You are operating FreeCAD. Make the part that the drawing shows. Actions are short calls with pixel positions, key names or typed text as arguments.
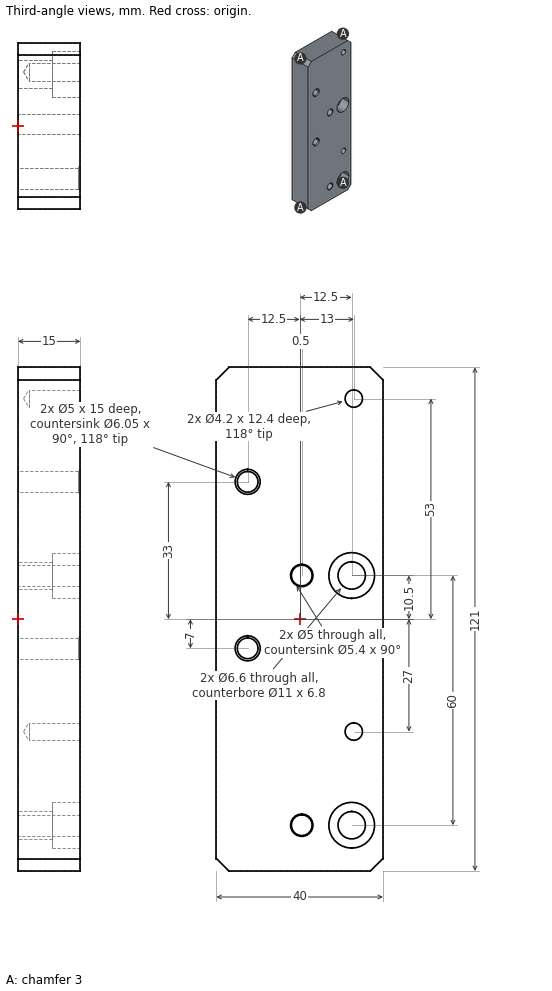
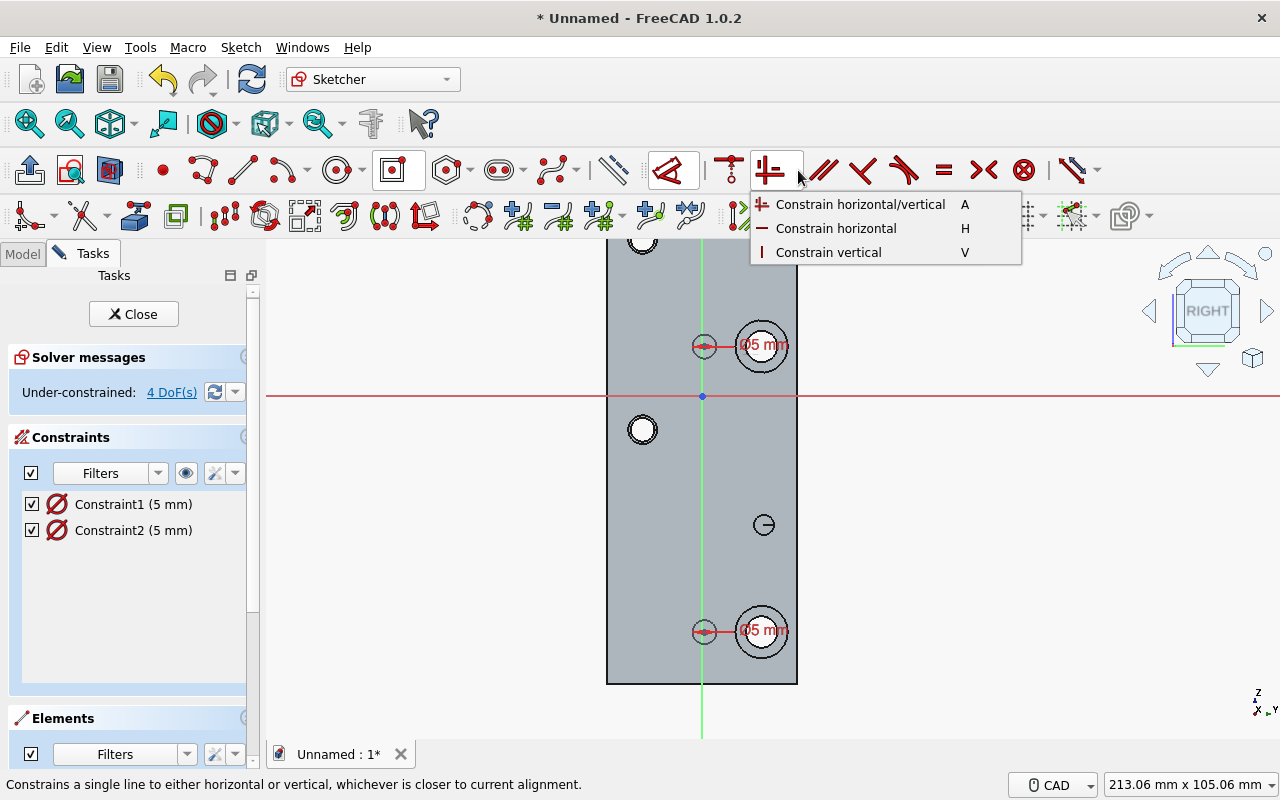
click(886, 252)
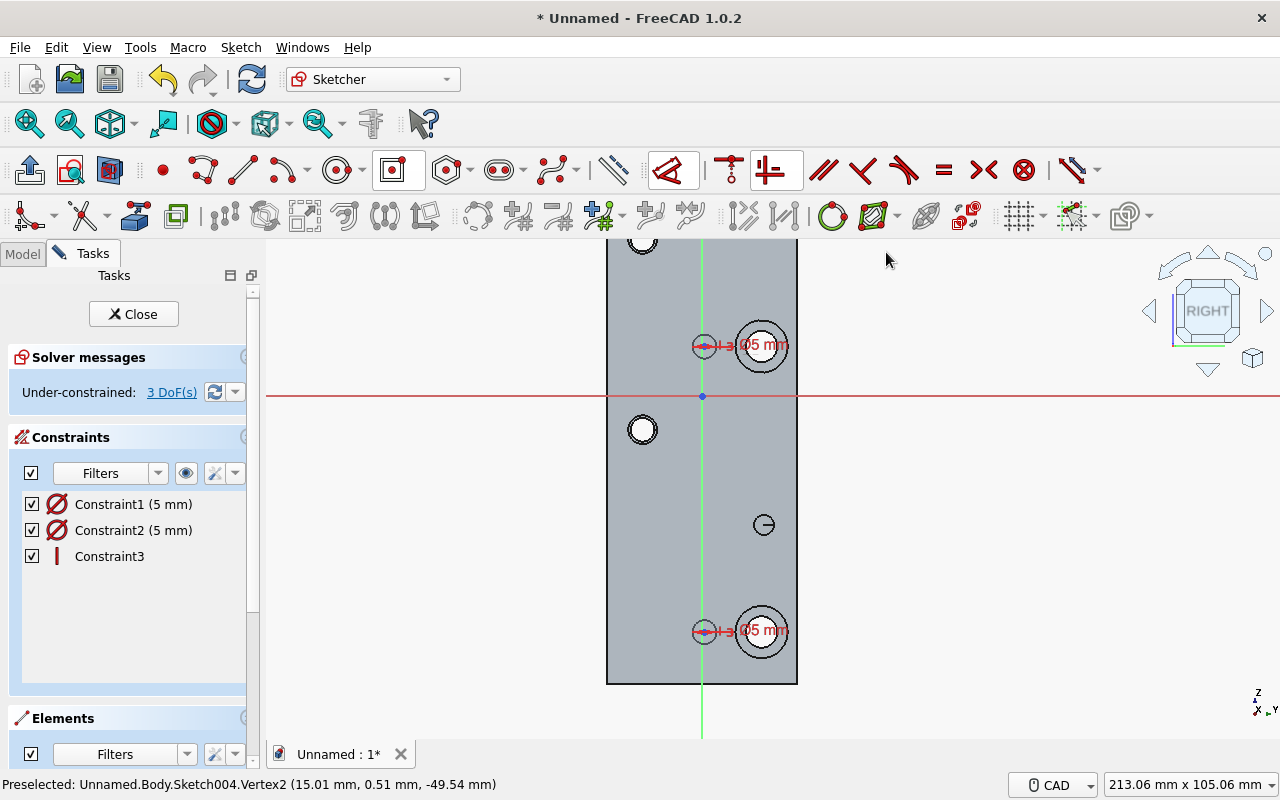
scroll(705, 347, up, 15)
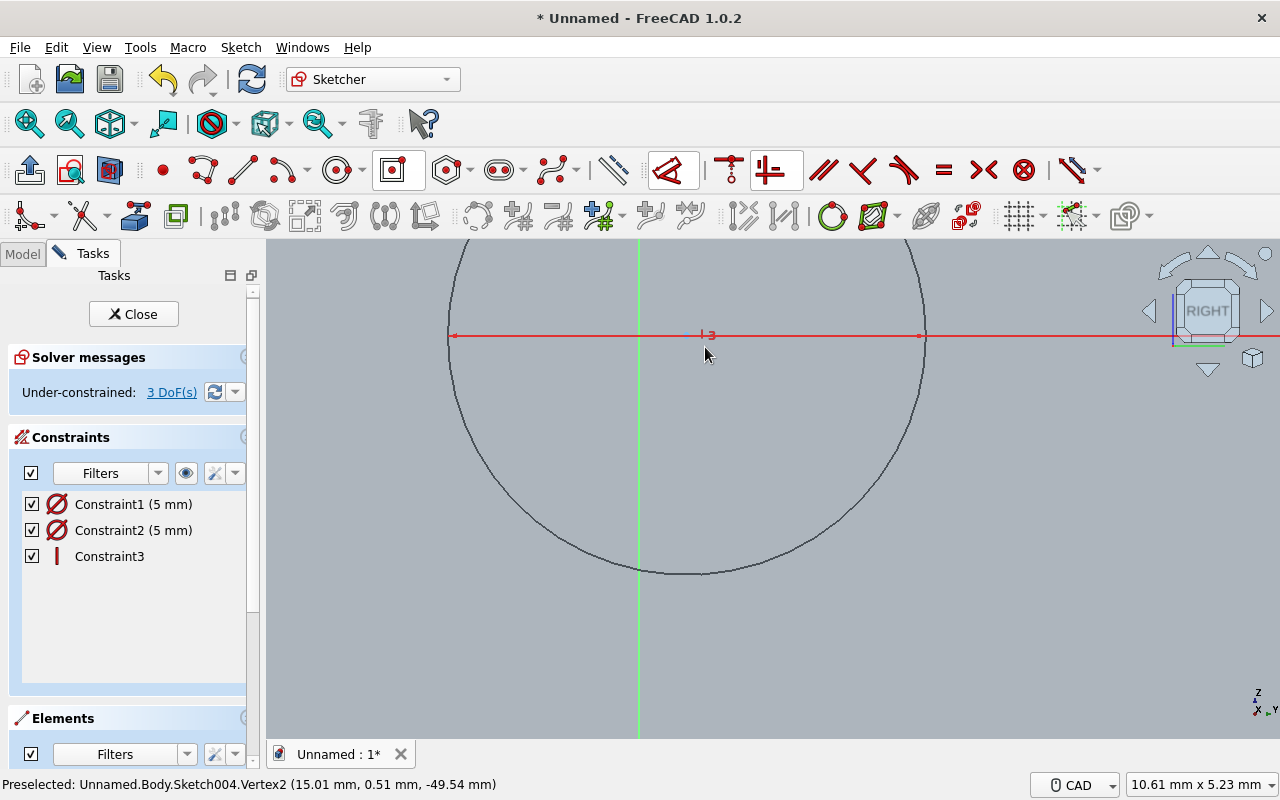
click(687, 336)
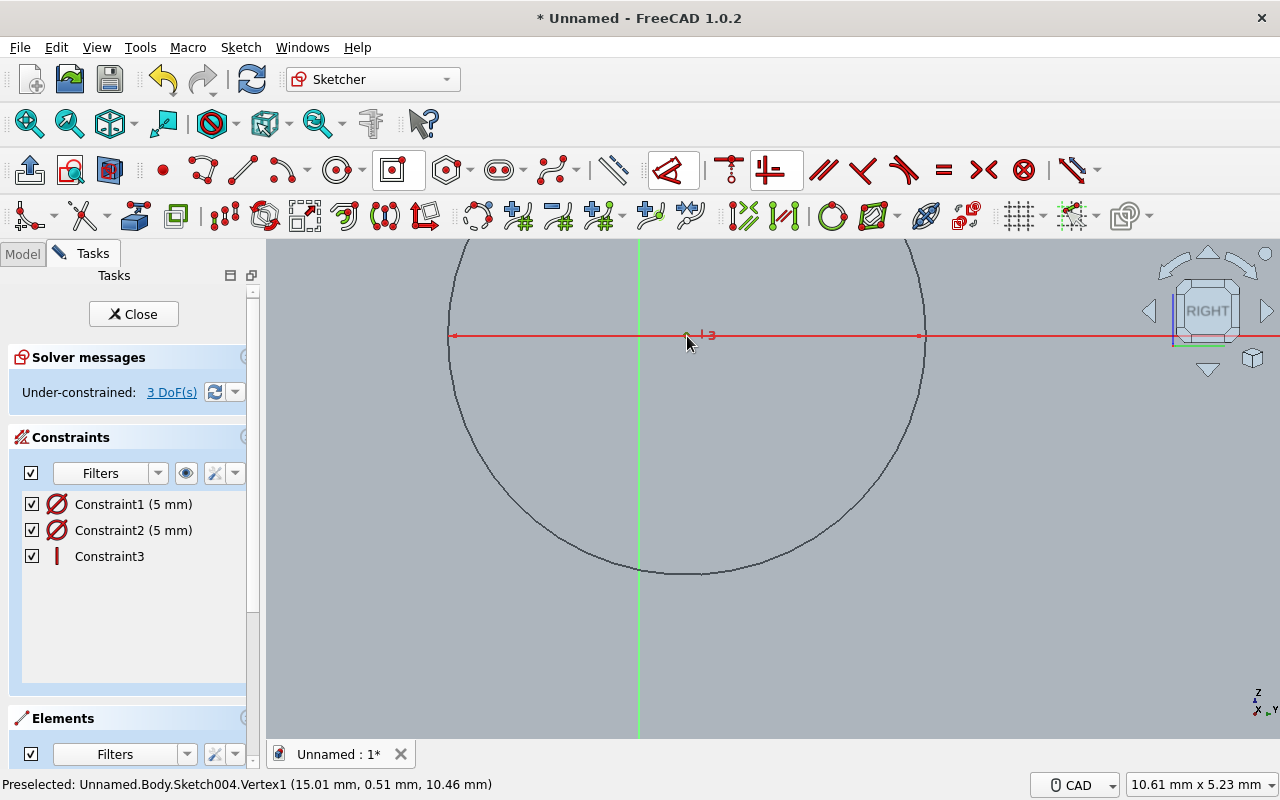
key(l)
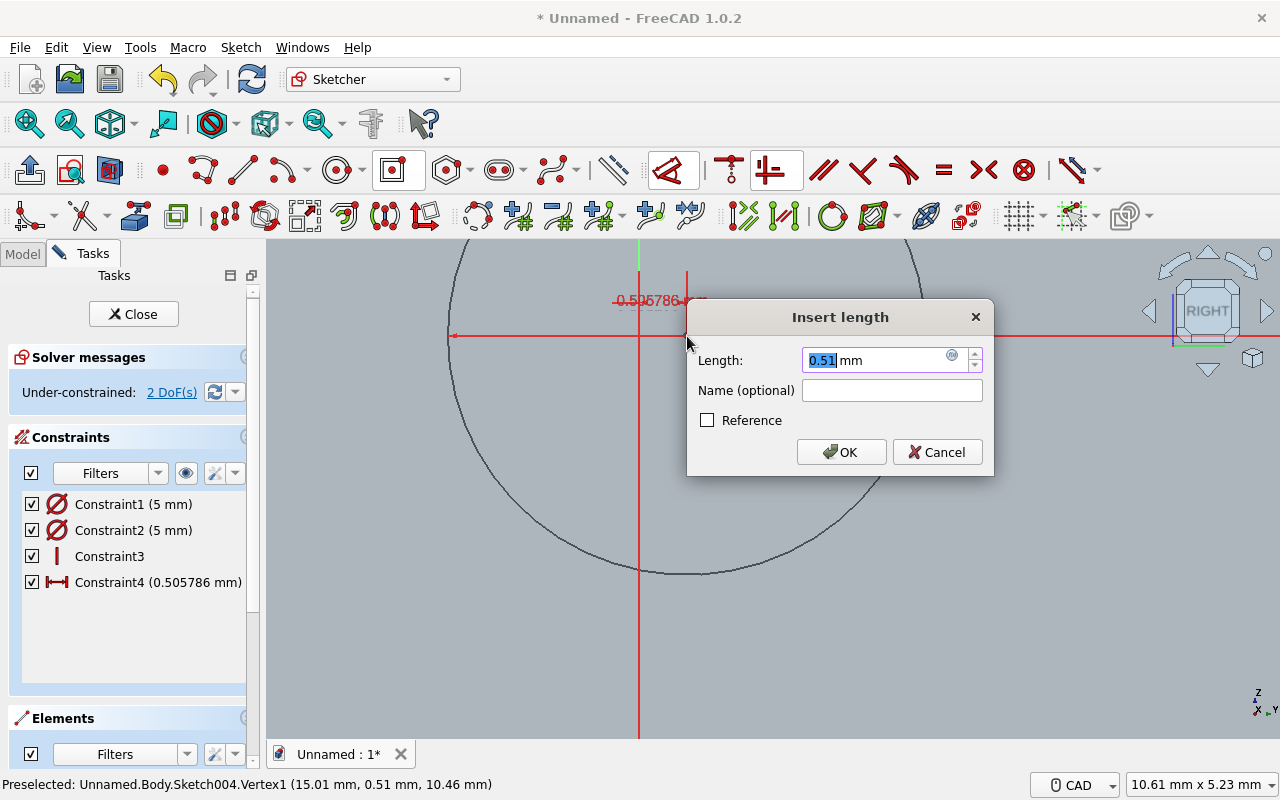
text(0.5)
key(Return)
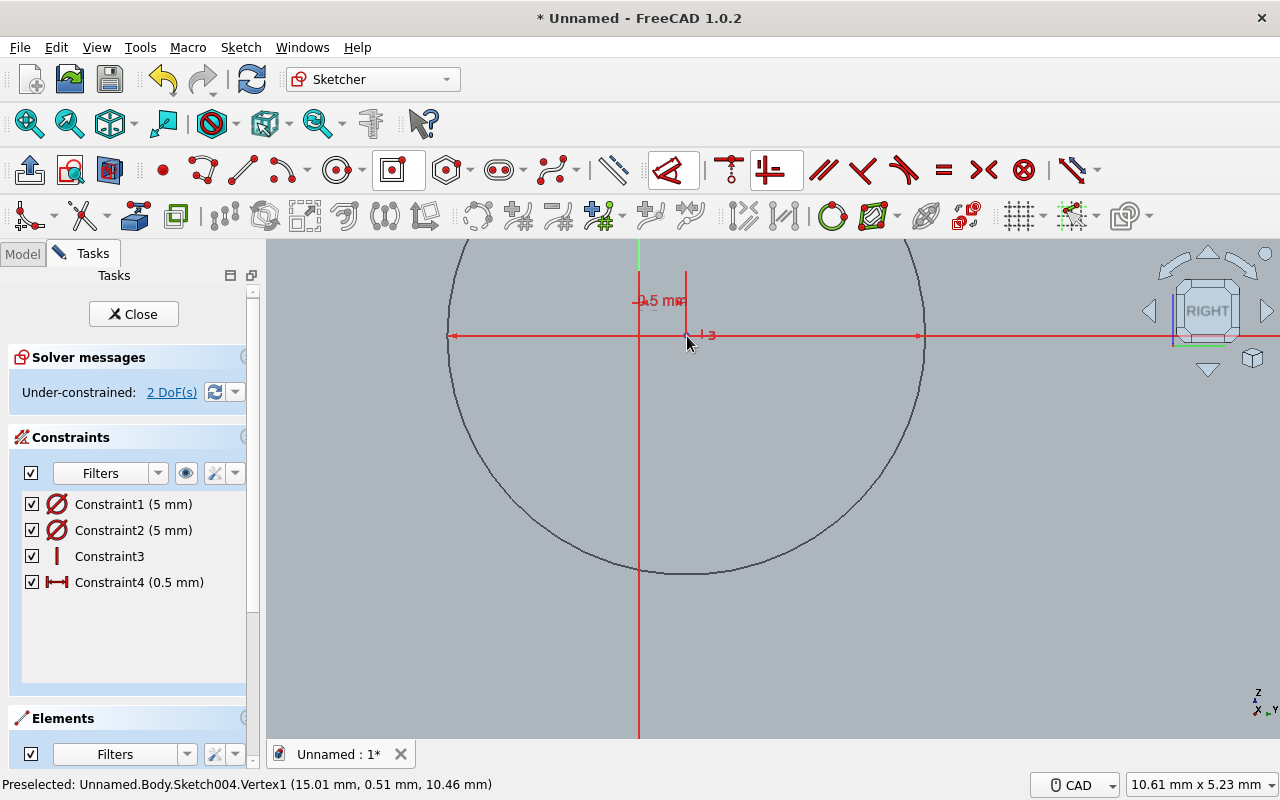
scroll(705, 347, down, 15)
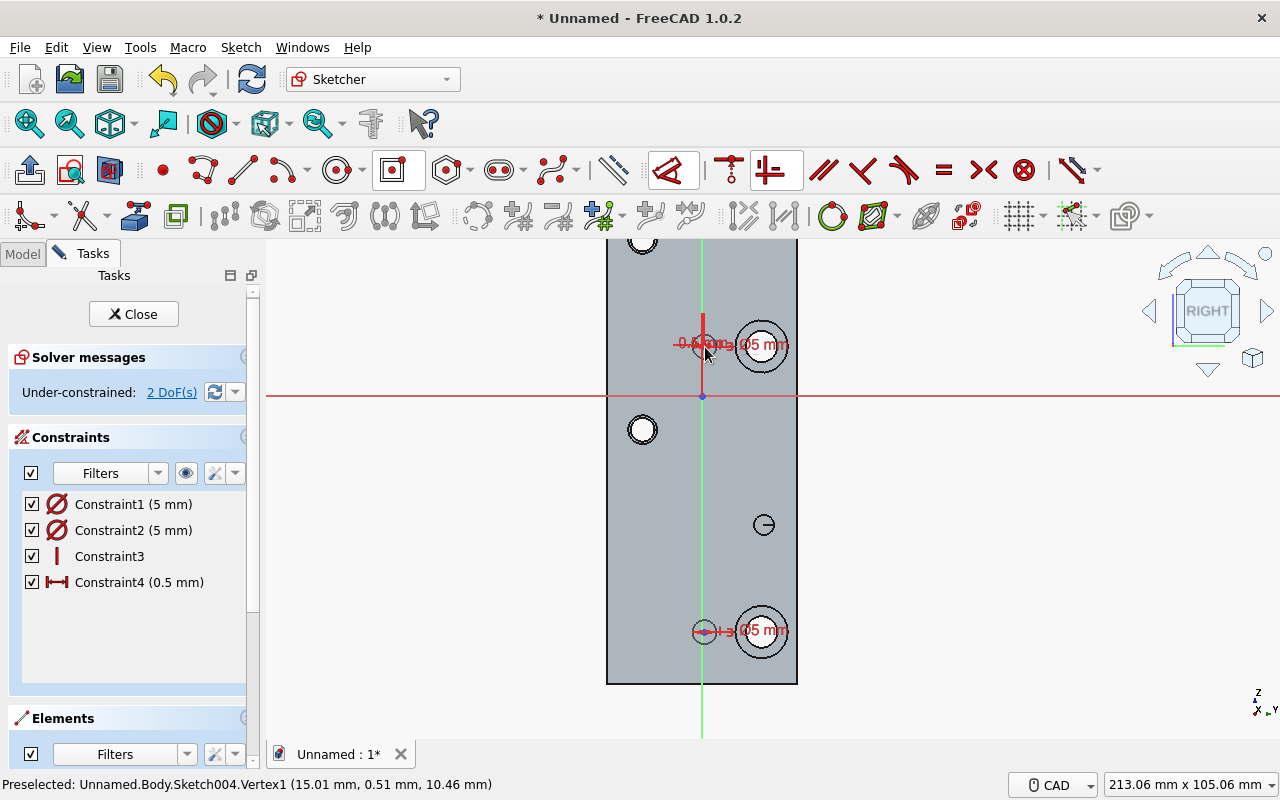
click(704, 347)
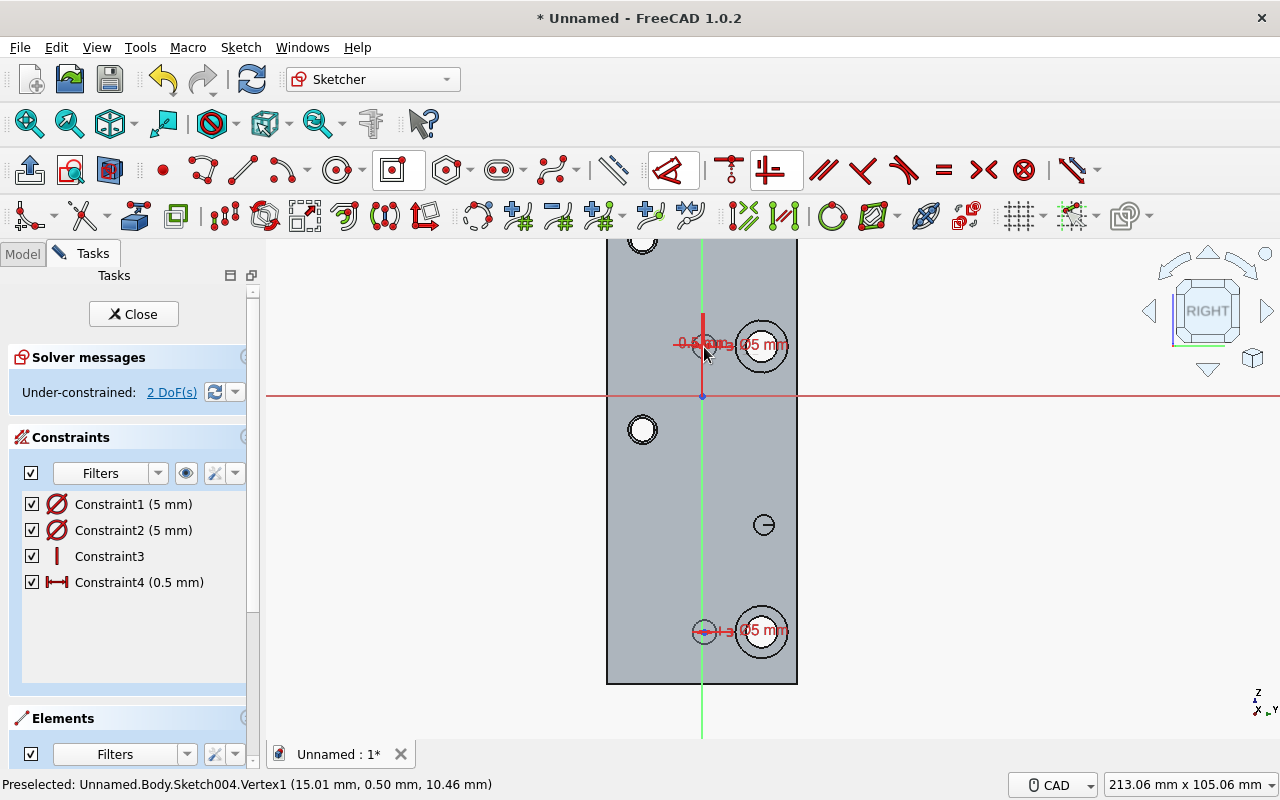
click(704, 632)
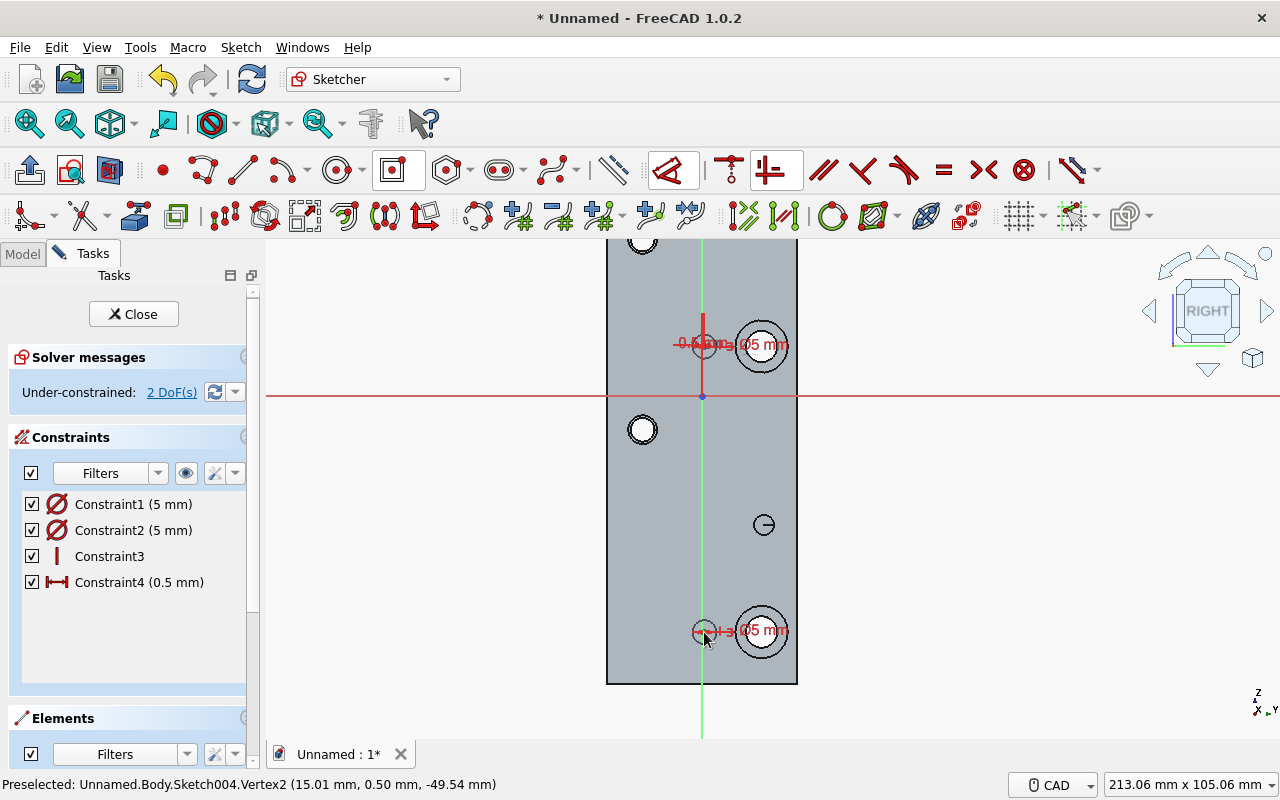
click(694, 170)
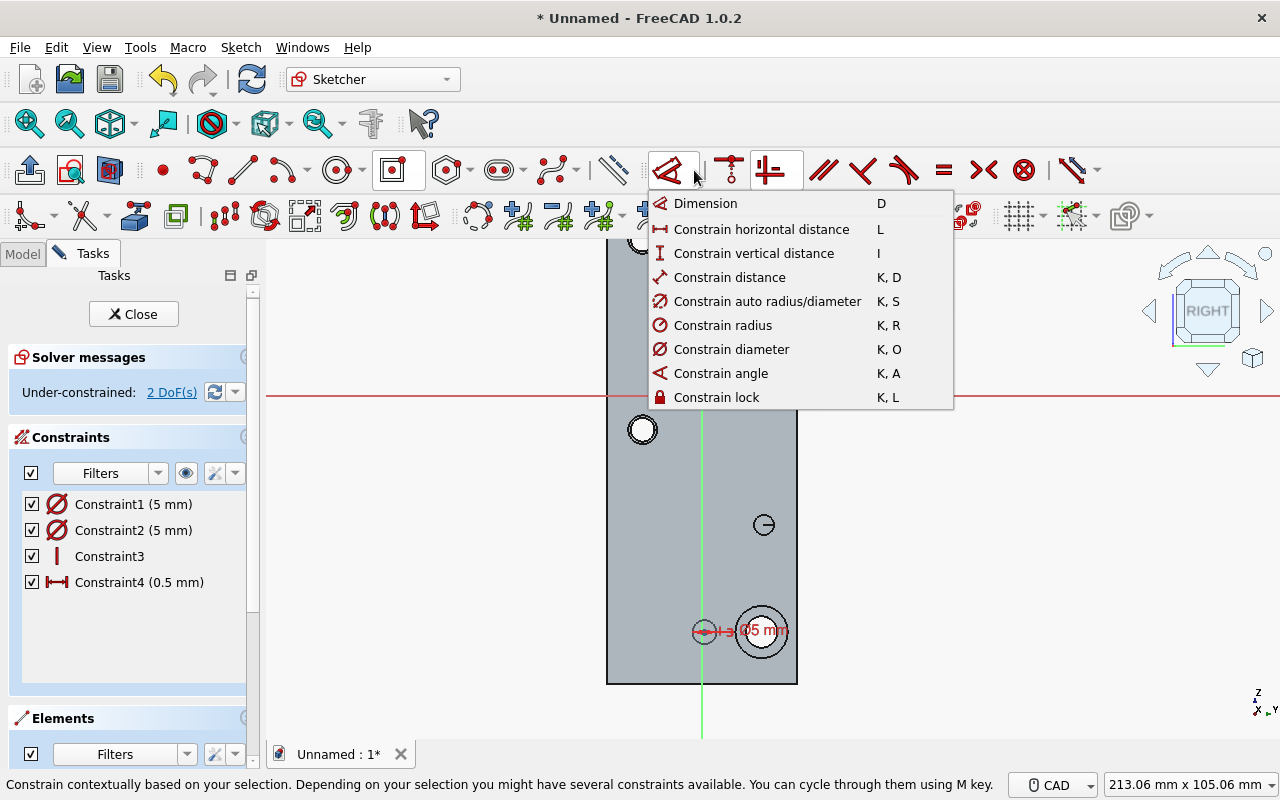
click(801, 253)